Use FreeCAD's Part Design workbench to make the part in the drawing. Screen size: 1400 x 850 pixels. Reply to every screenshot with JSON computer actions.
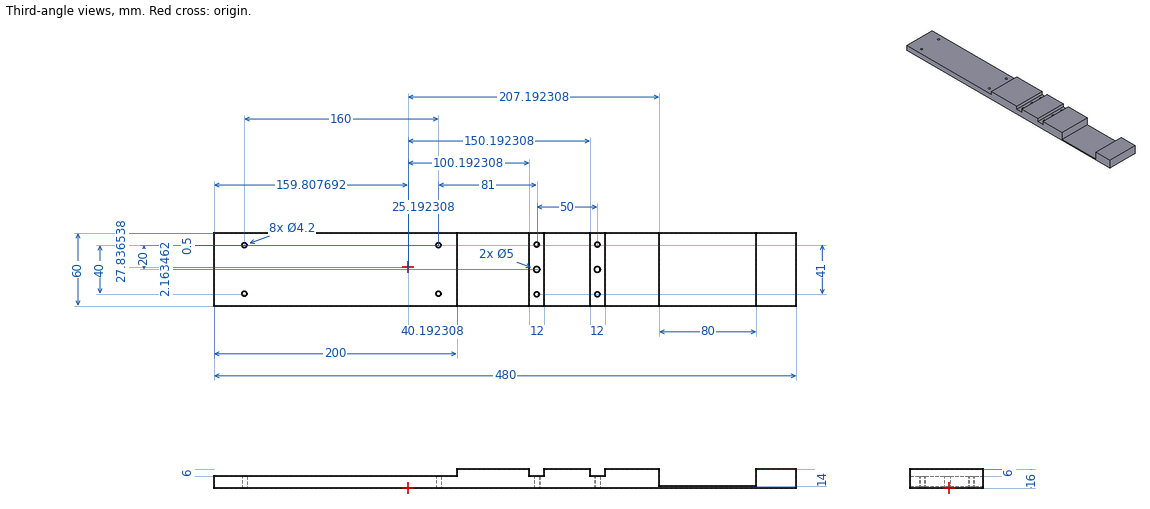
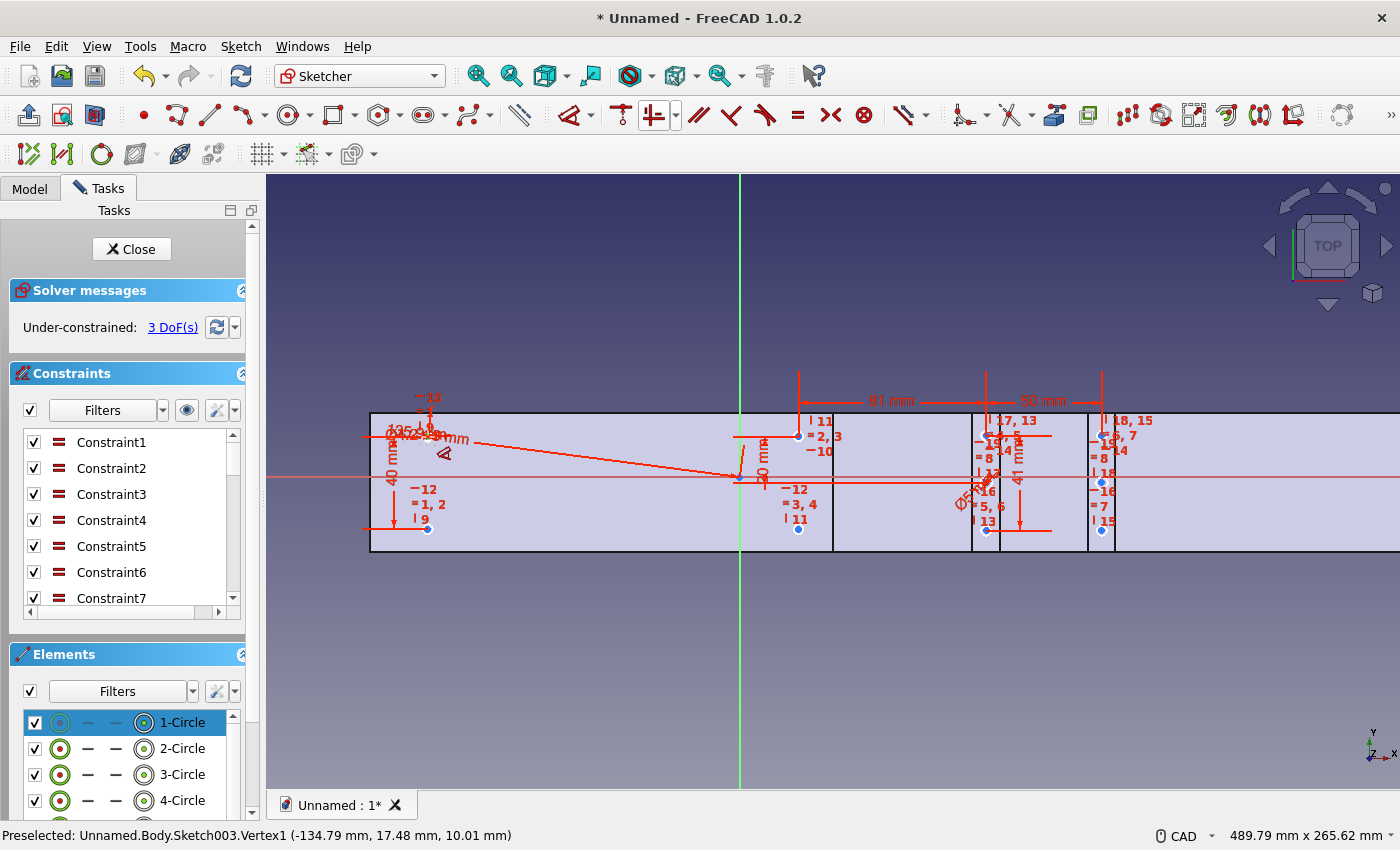
{"action": "left_click", "coordinate": [799, 437]}
{"action": "left_click", "coordinate": [613, 403]}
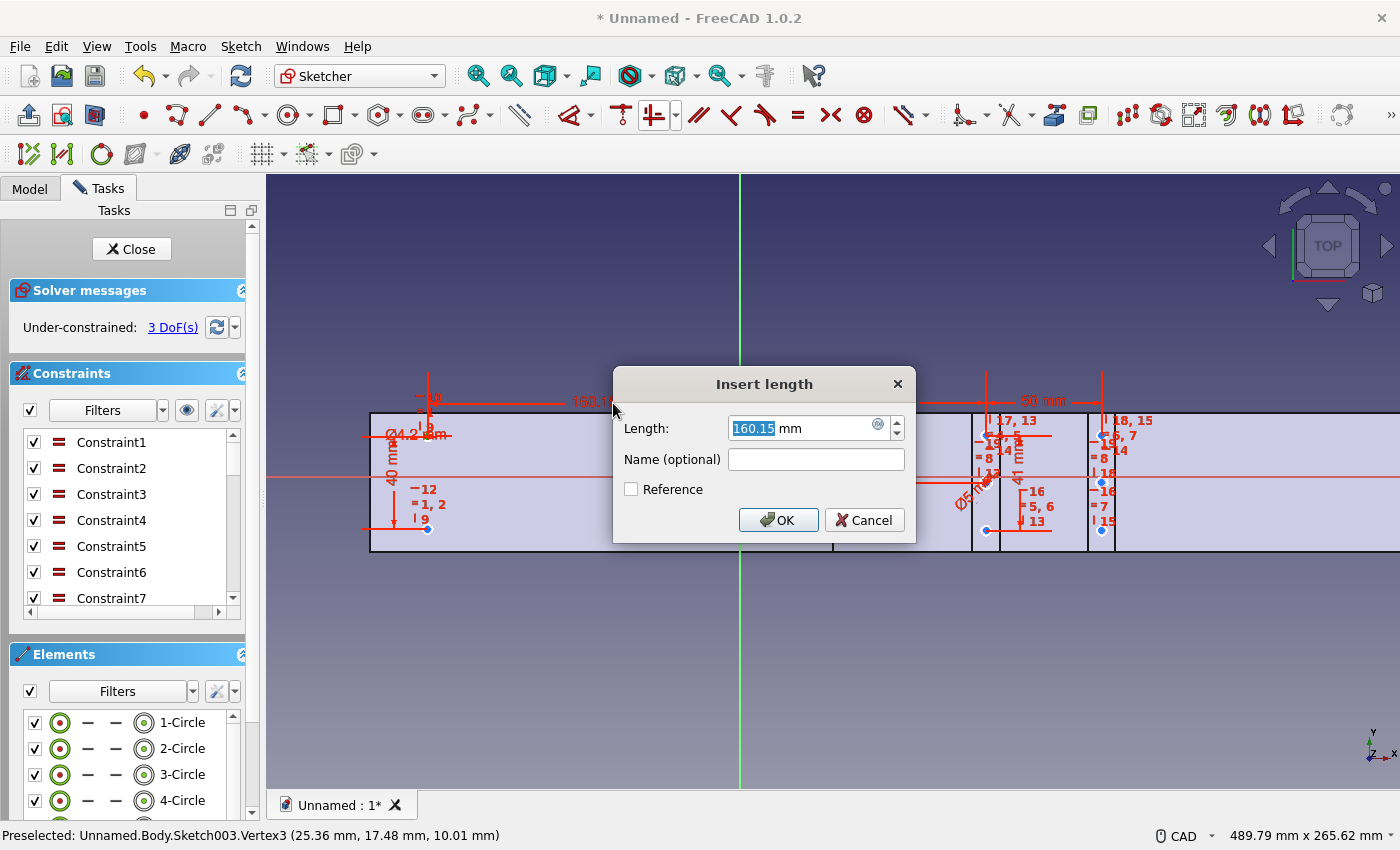
{"action": "type", "text": "160"}
{"action": "key", "text": "Return"}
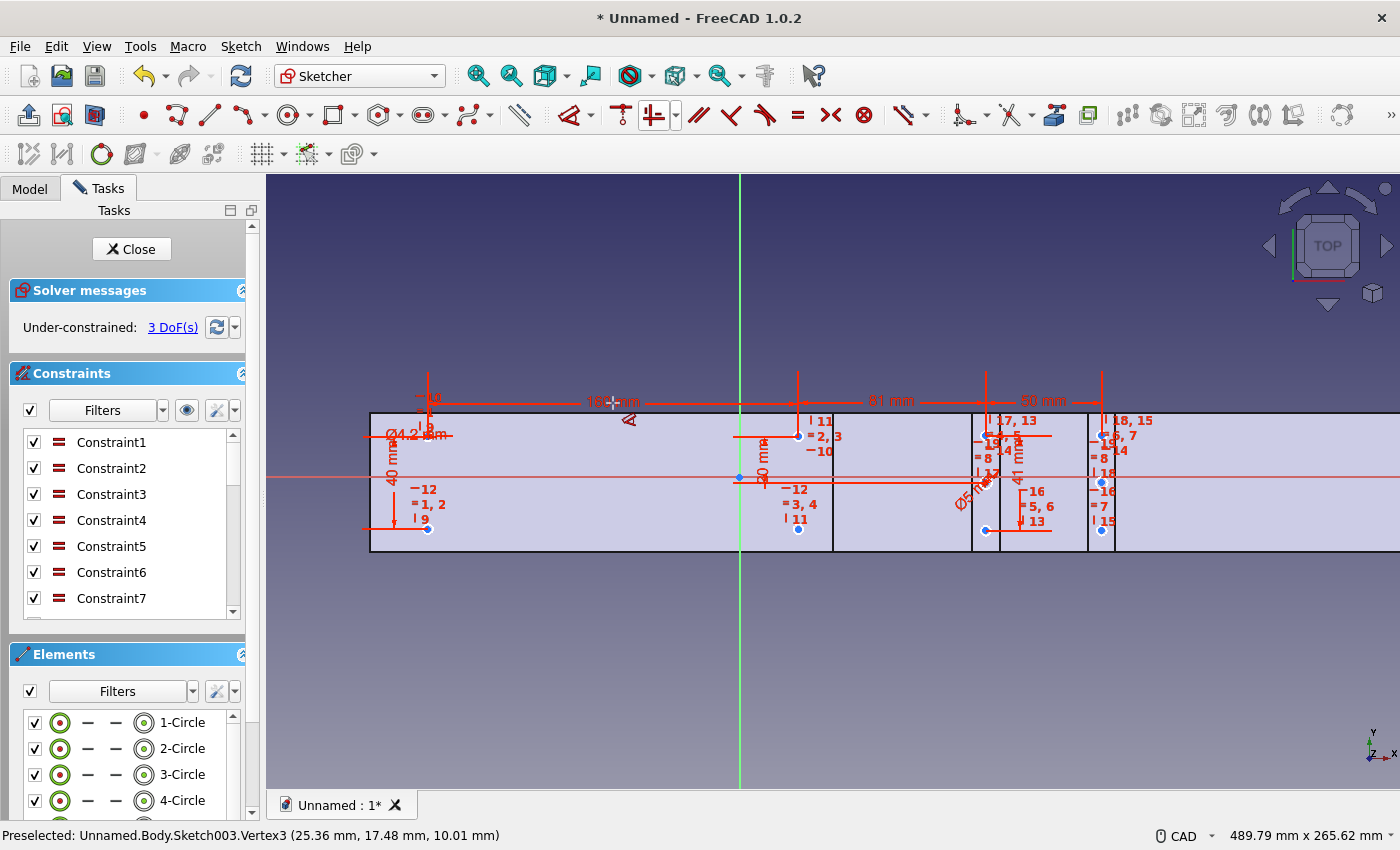
{"action": "scroll", "coordinate": [798, 437], "scroll_direction": "up", "scroll_amount": 18}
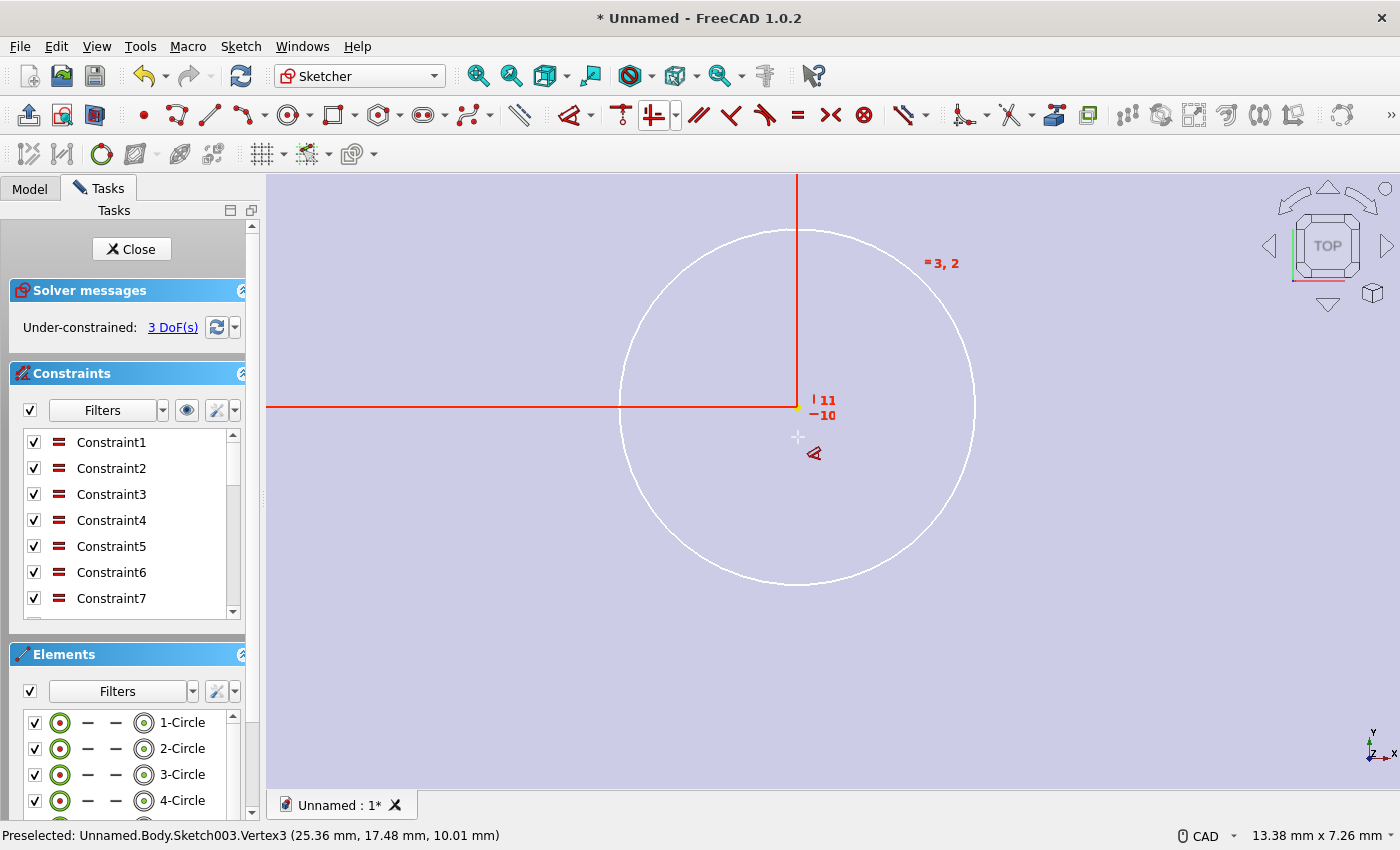
{"action": "left_click", "coordinate": [797, 407]}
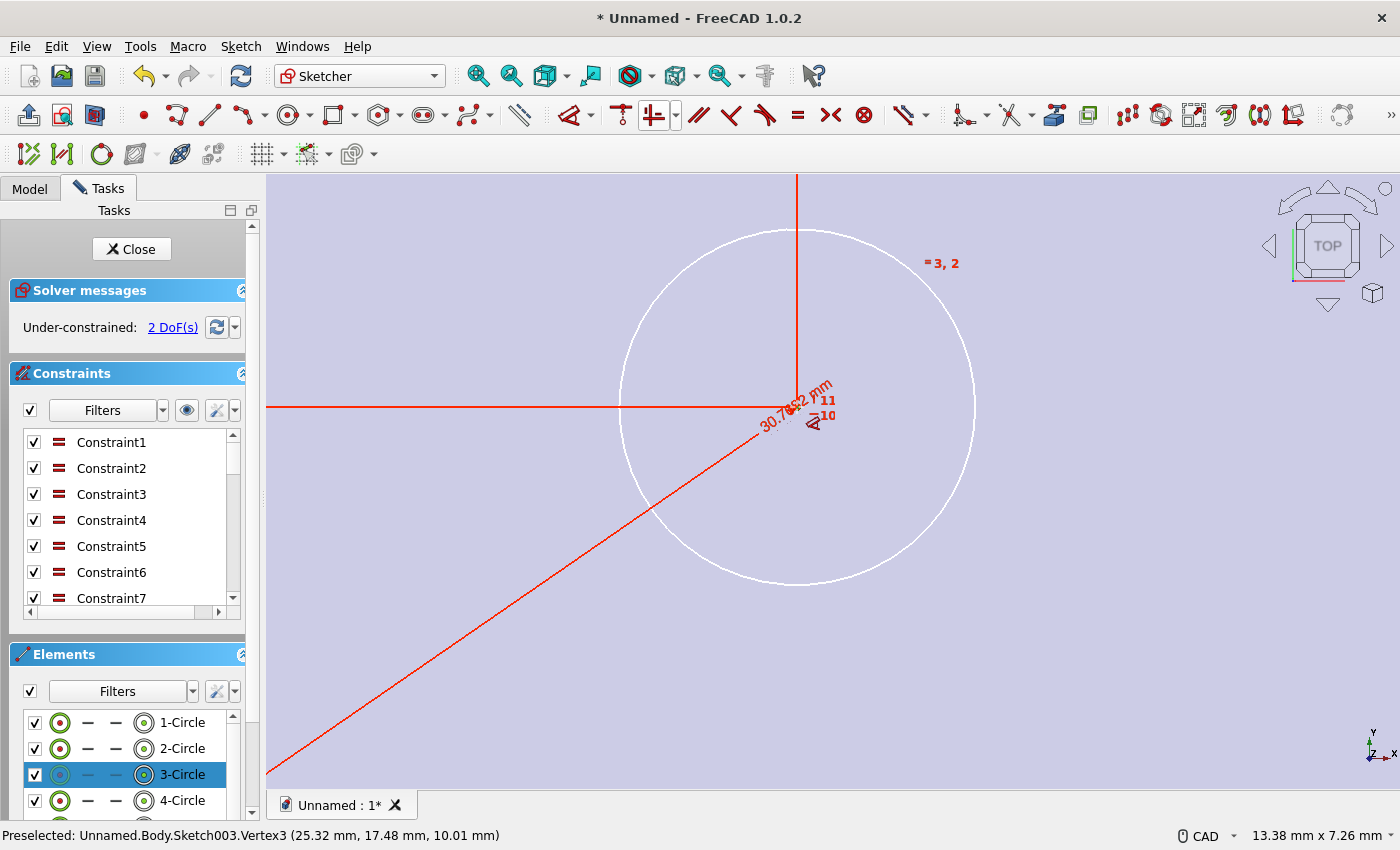
{"action": "scroll", "coordinate": [806, 427], "scroll_direction": "down", "scroll_amount": 17}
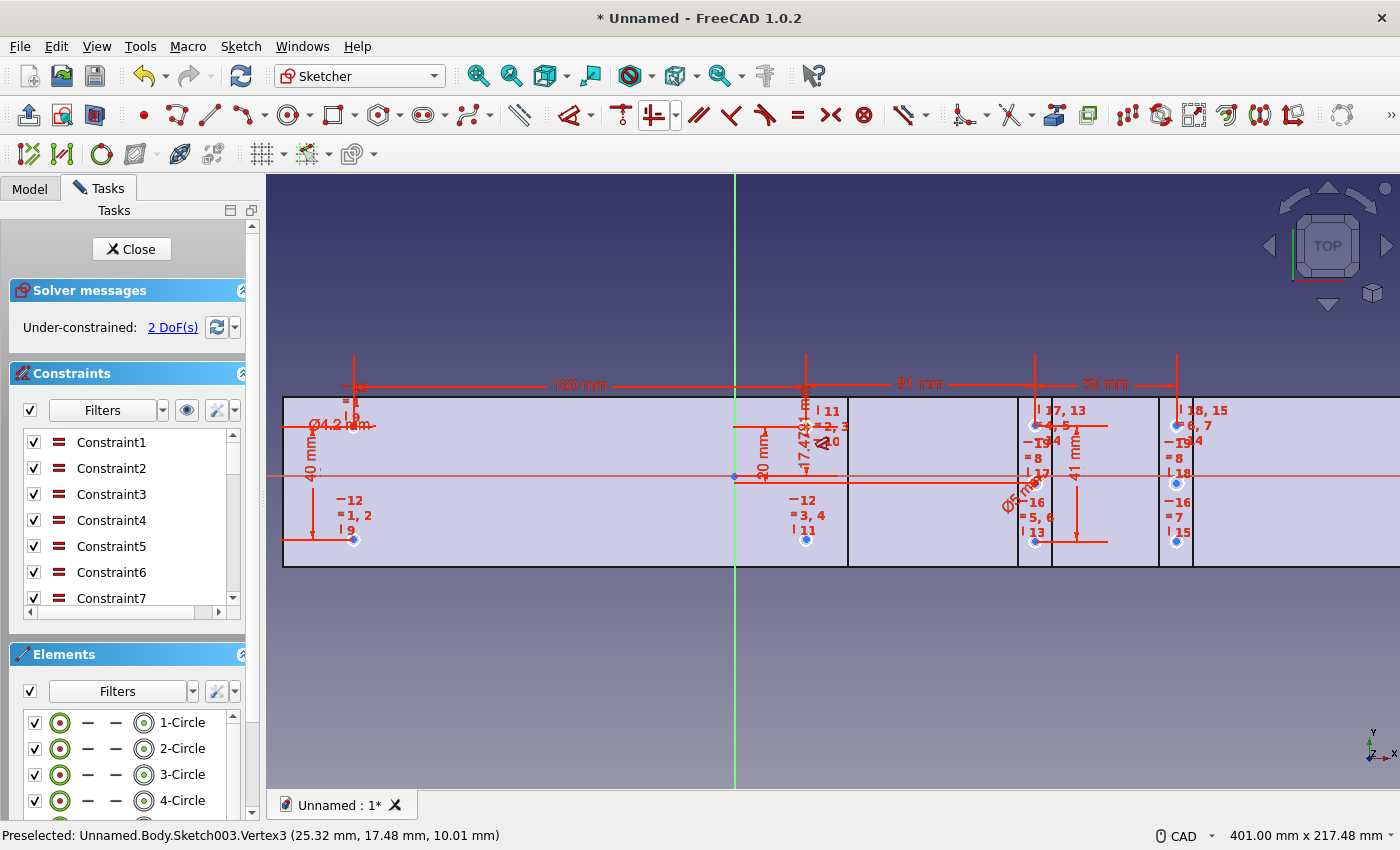
{"action": "scroll", "coordinate": [1035, 426], "scroll_direction": "up", "scroll_amount": 17}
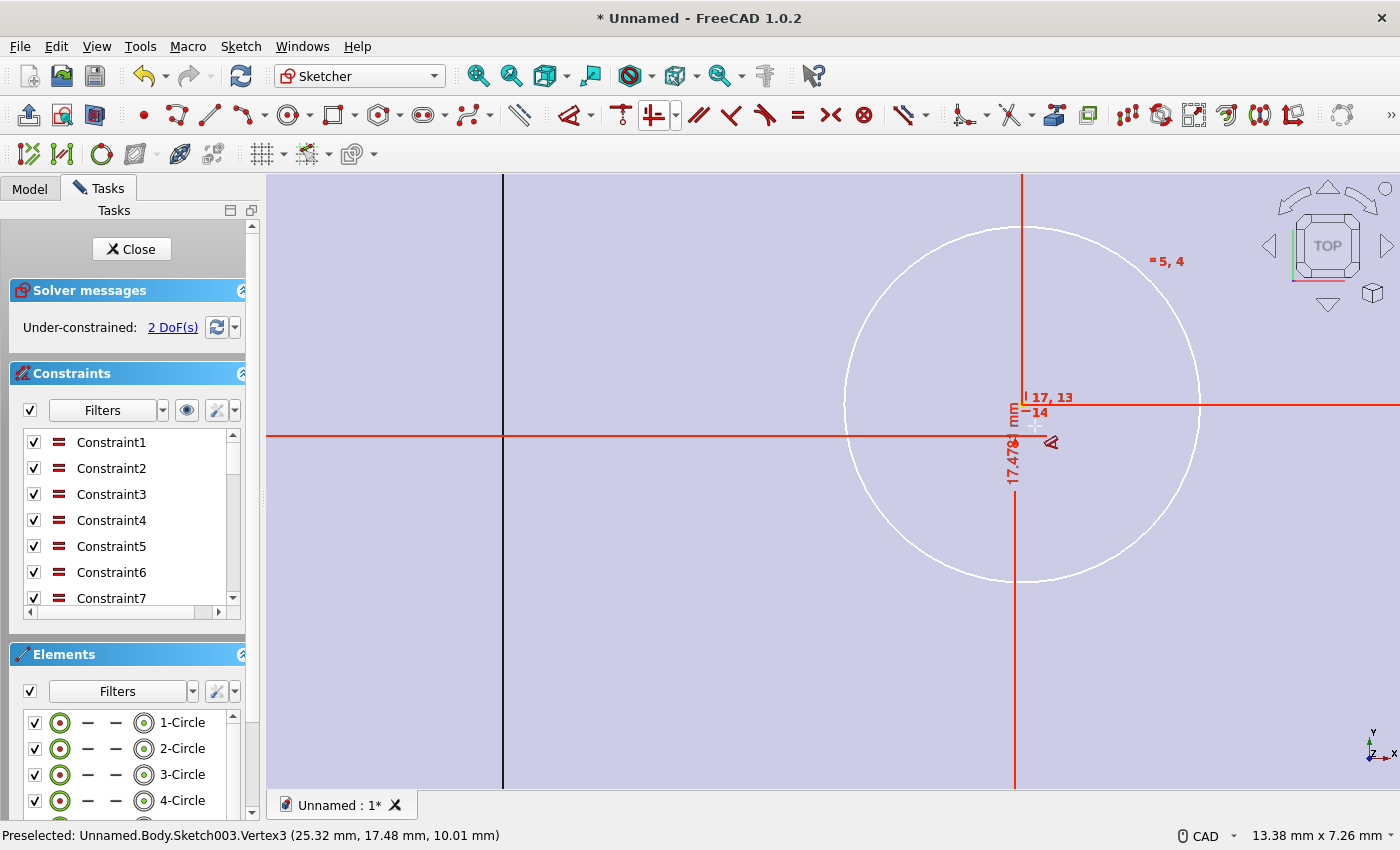
{"action": "left_click", "coordinate": [1022, 405]}
{"action": "left_click", "coordinate": [1056, 420]}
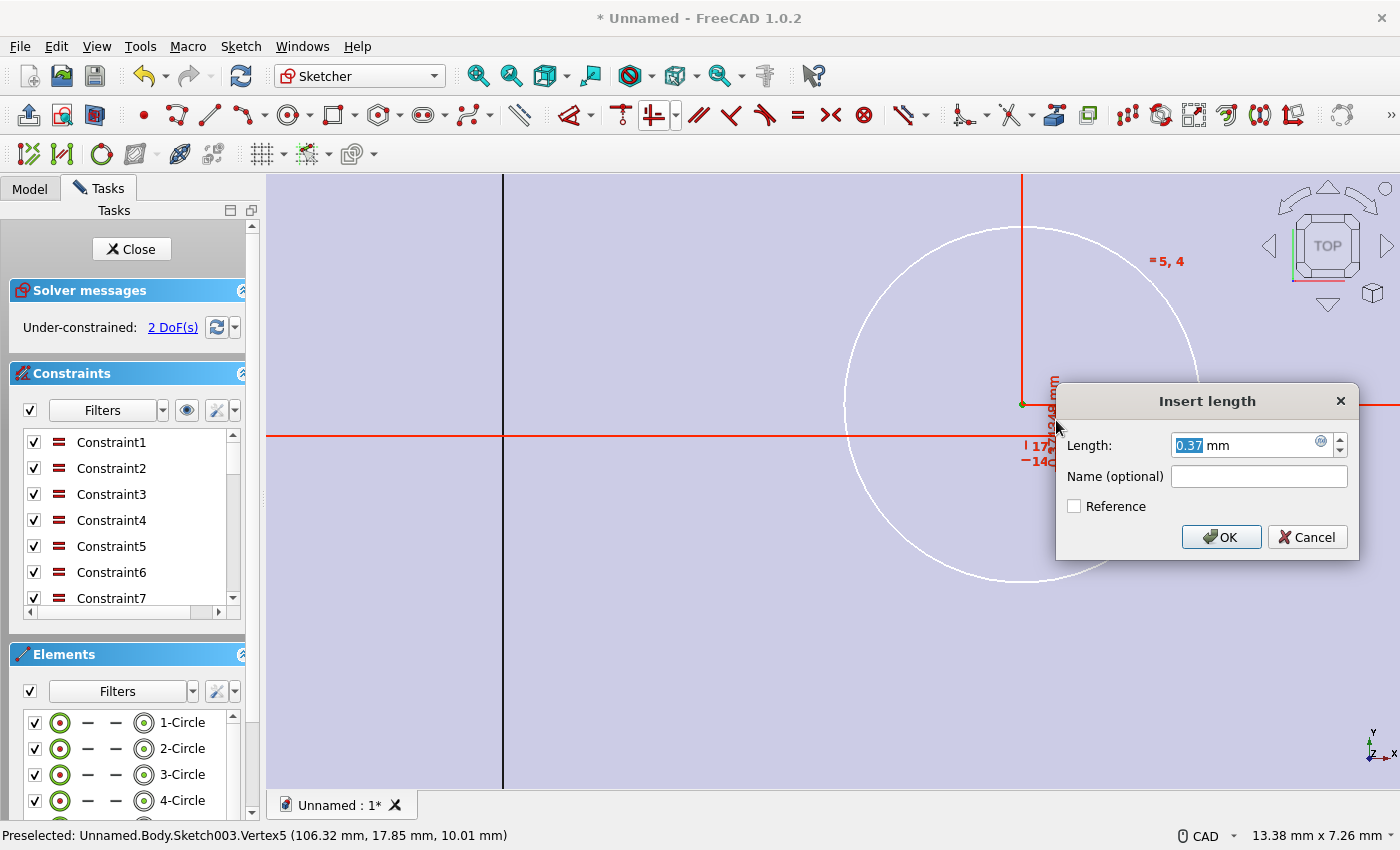
{"action": "type", "text": "0.5"}
{"action": "key", "text": "Return"}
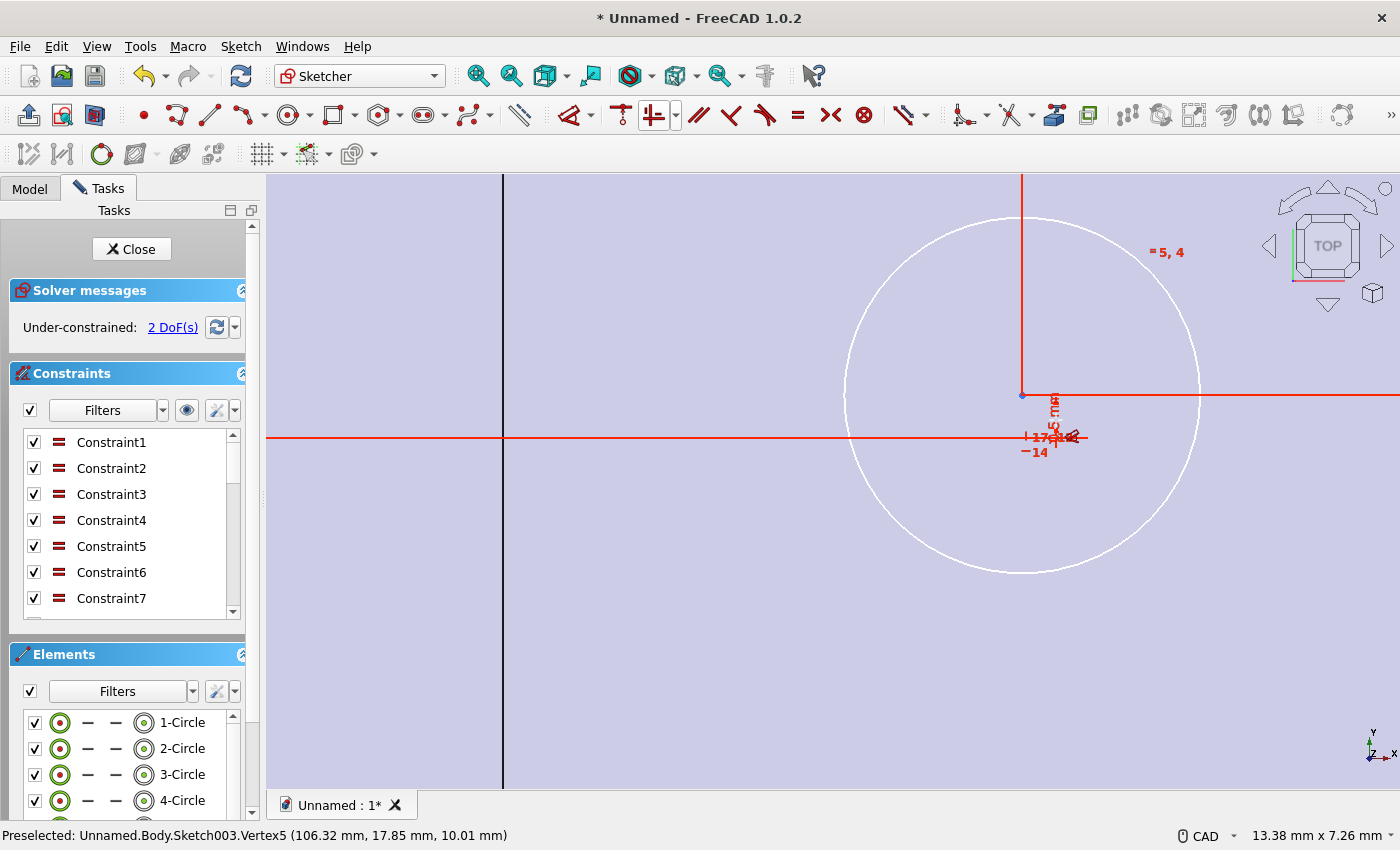
{"action": "scroll", "coordinate": [1035, 426], "scroll_direction": "down", "scroll_amount": 17}